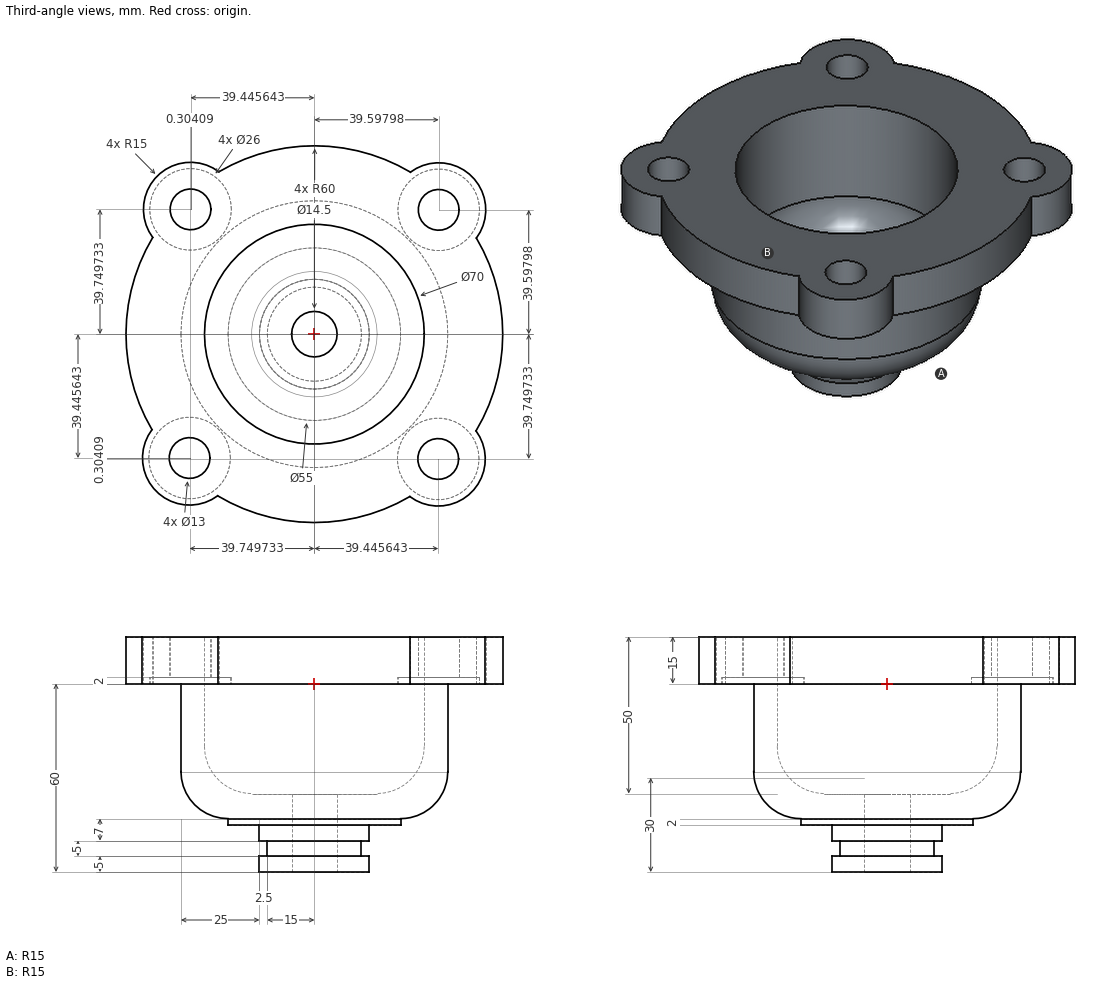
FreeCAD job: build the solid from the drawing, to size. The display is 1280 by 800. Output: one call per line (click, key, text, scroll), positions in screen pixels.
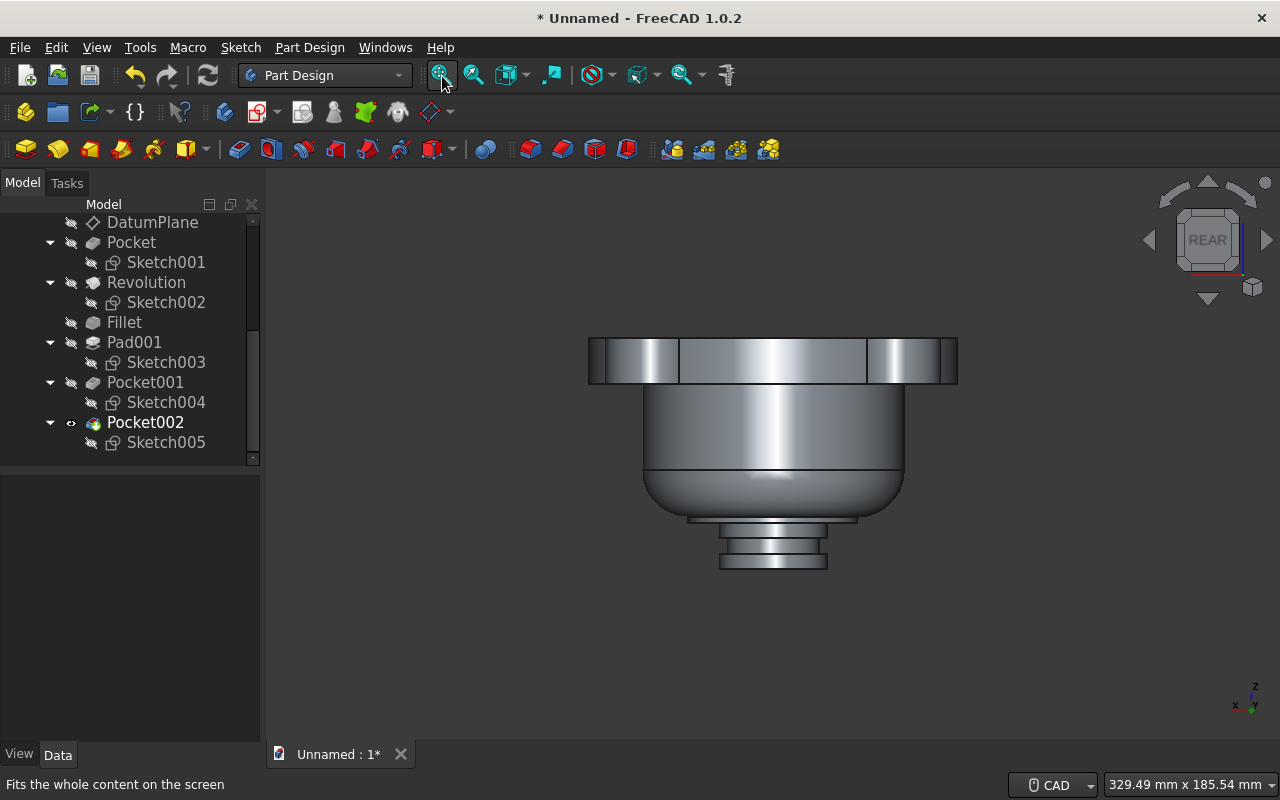
key(6)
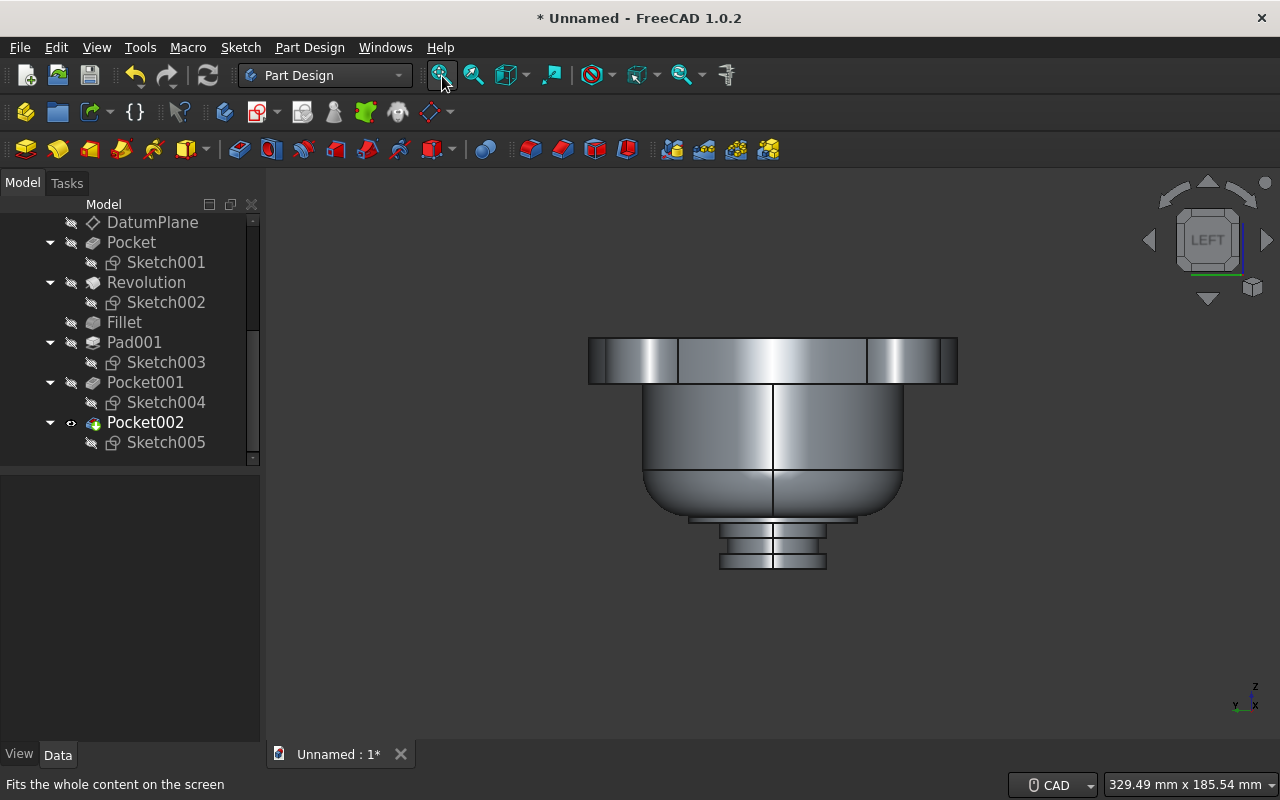
click(442, 76)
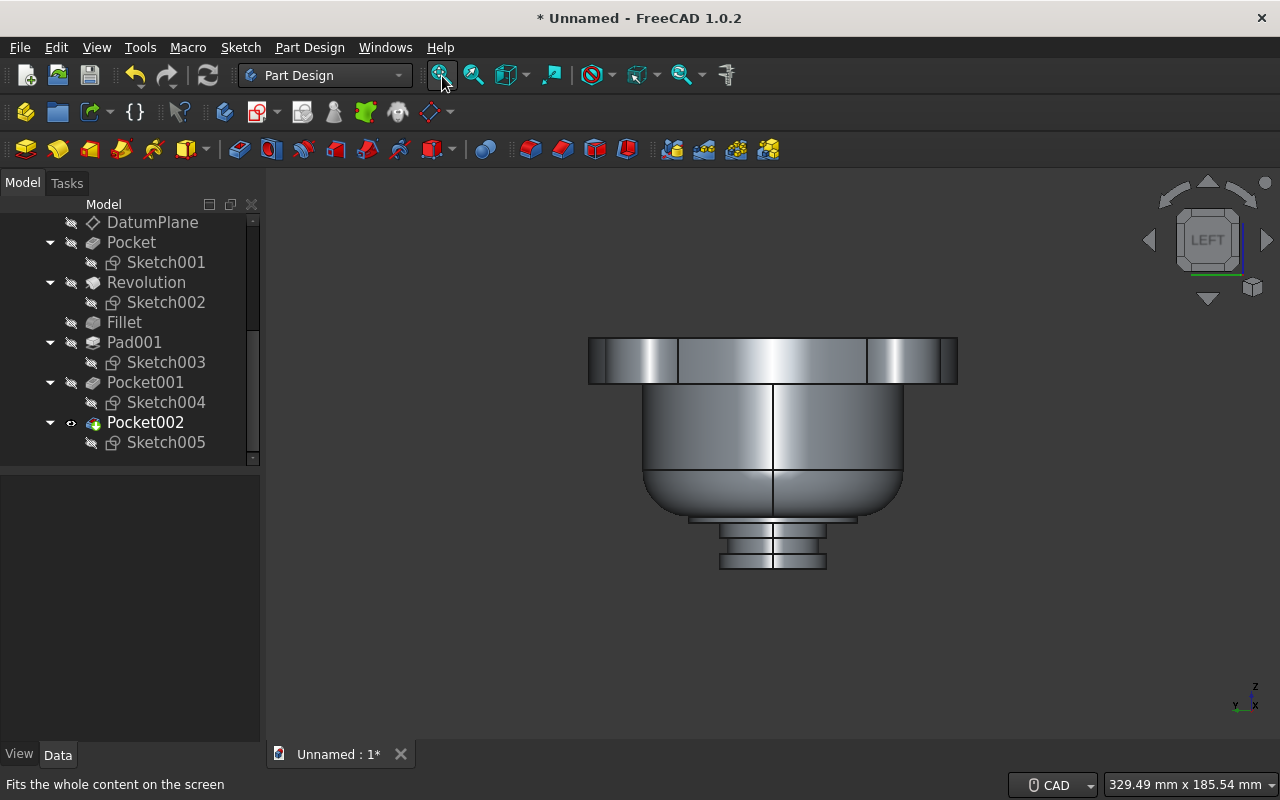
key(v)
key(3)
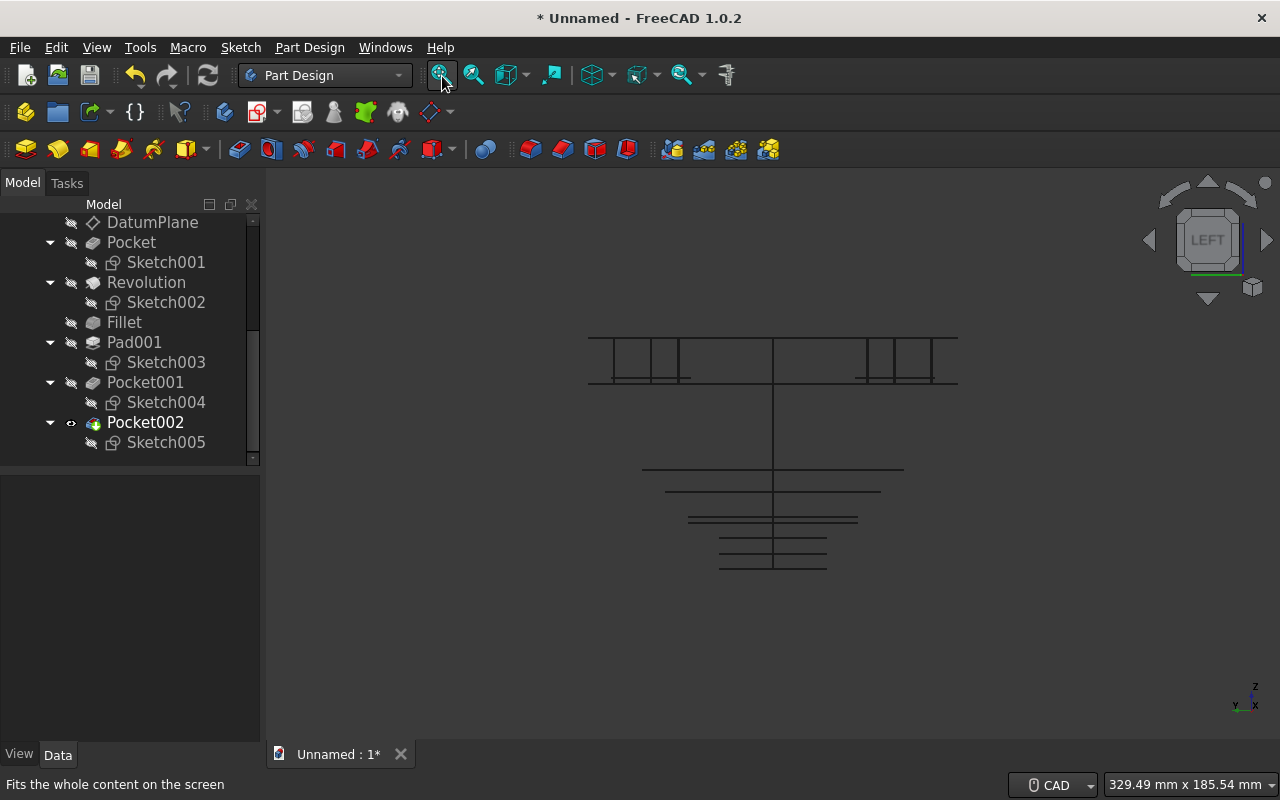
key(0)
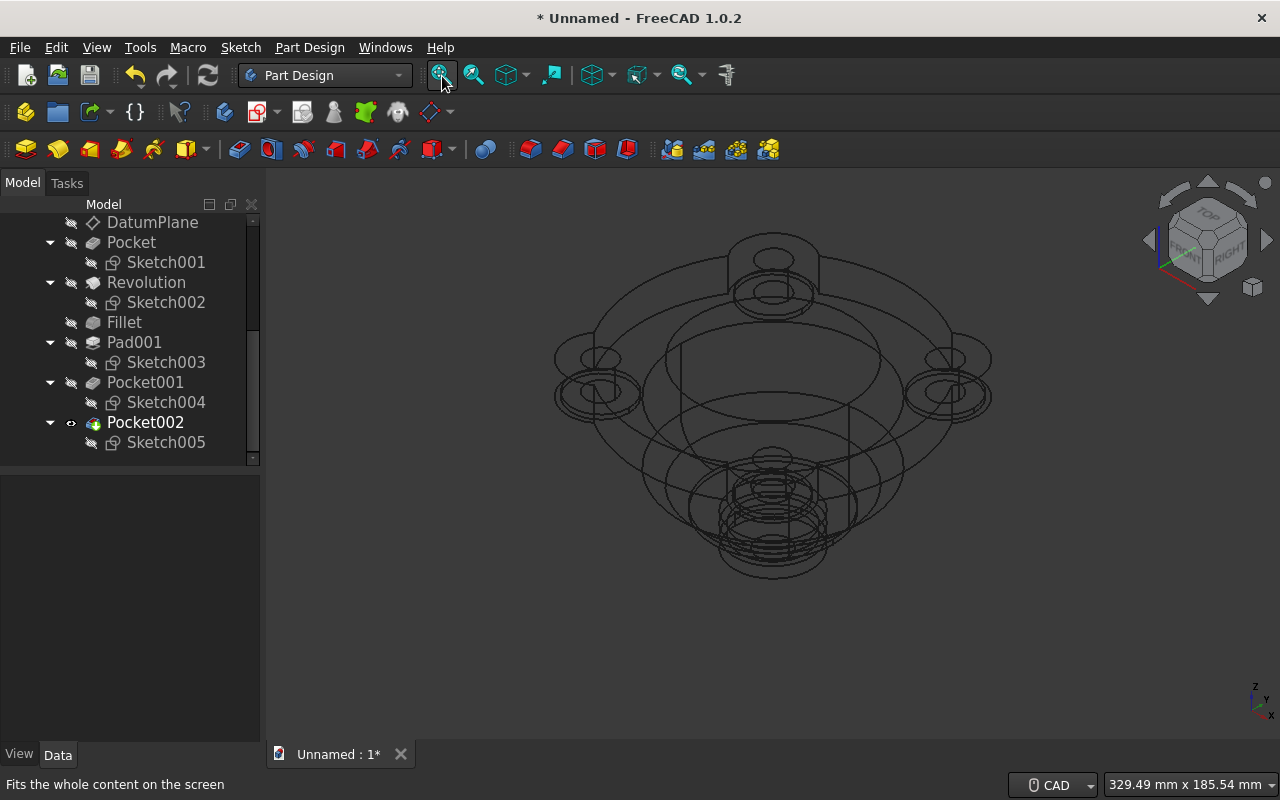
click(697, 440)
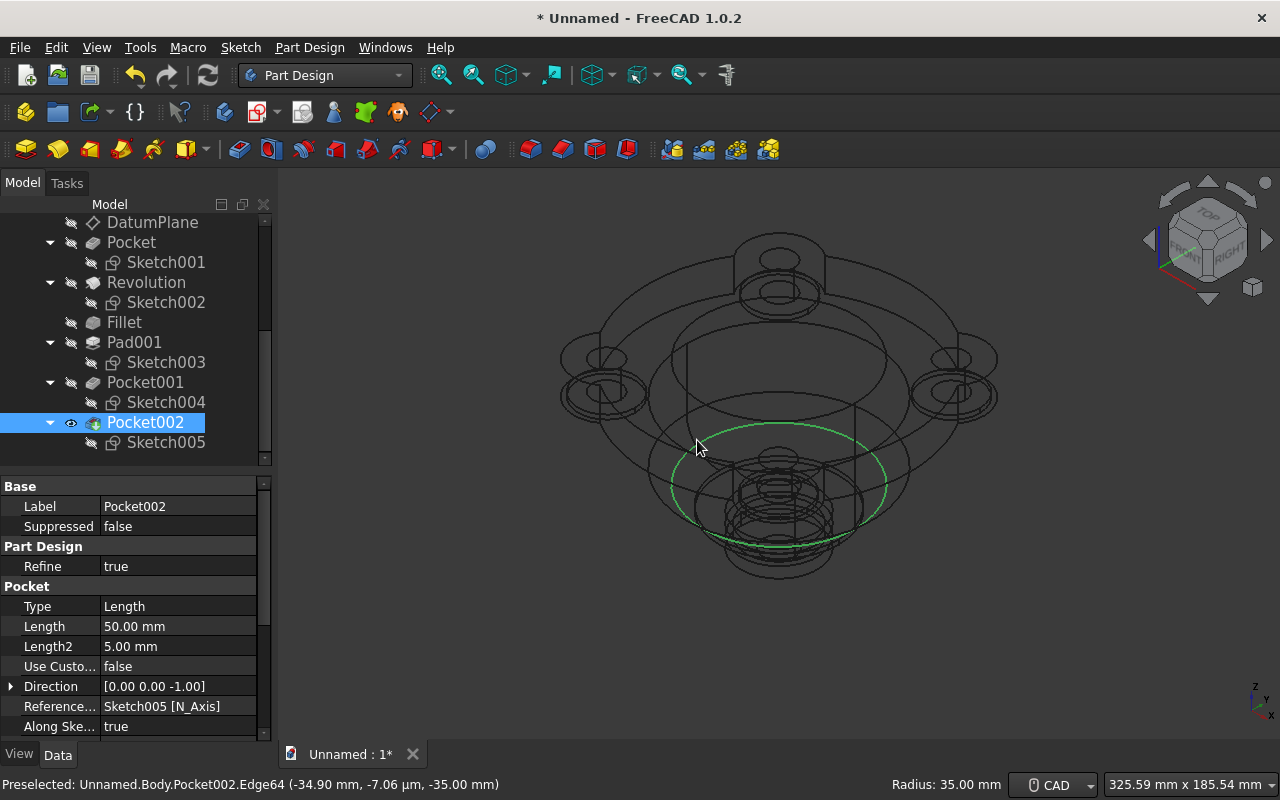
key(v)
key(1)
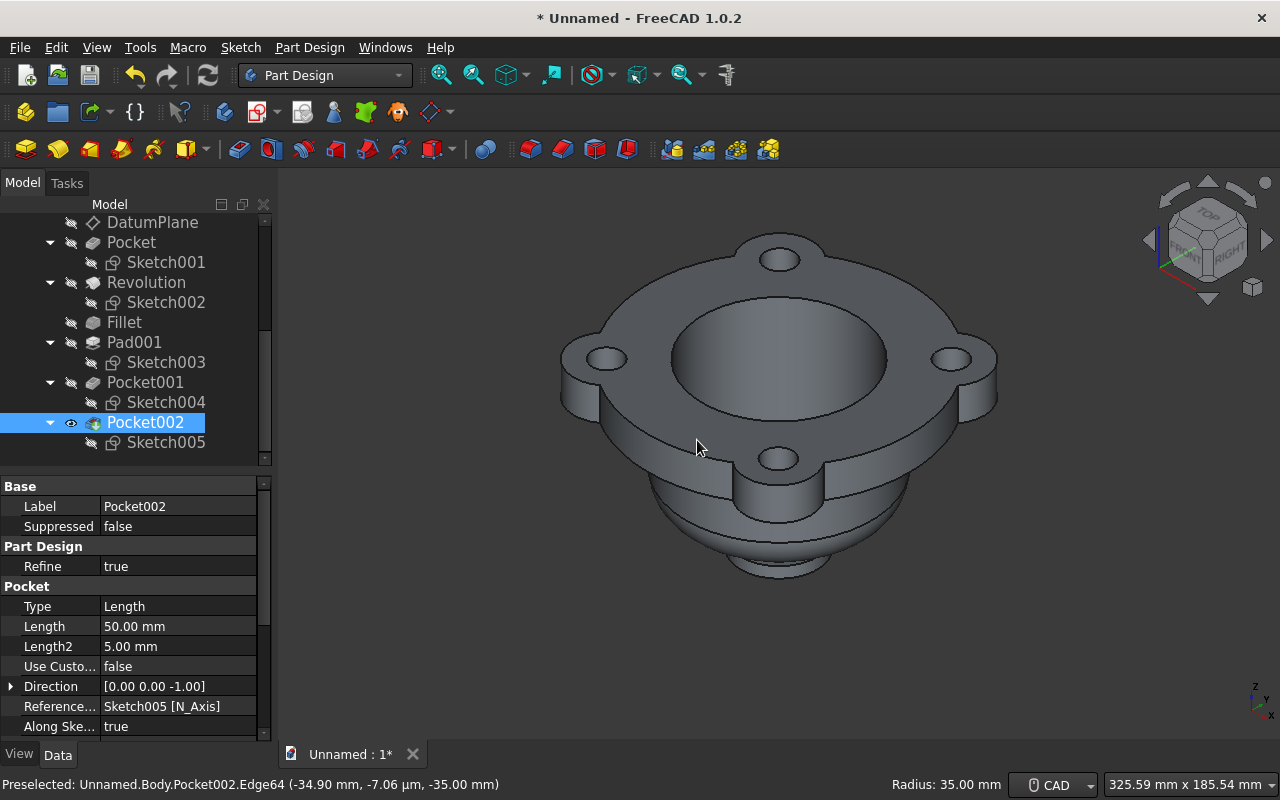
click(532, 150)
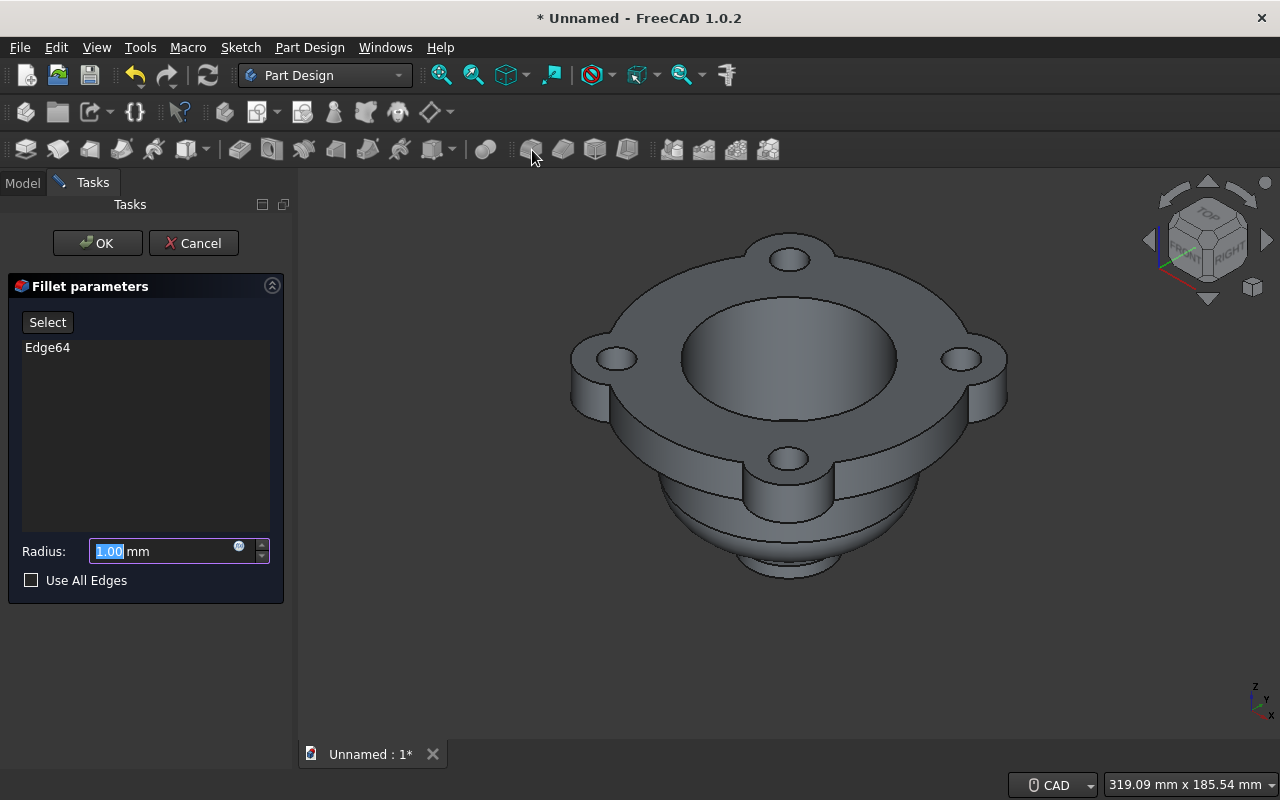
text(15)
key(Tab)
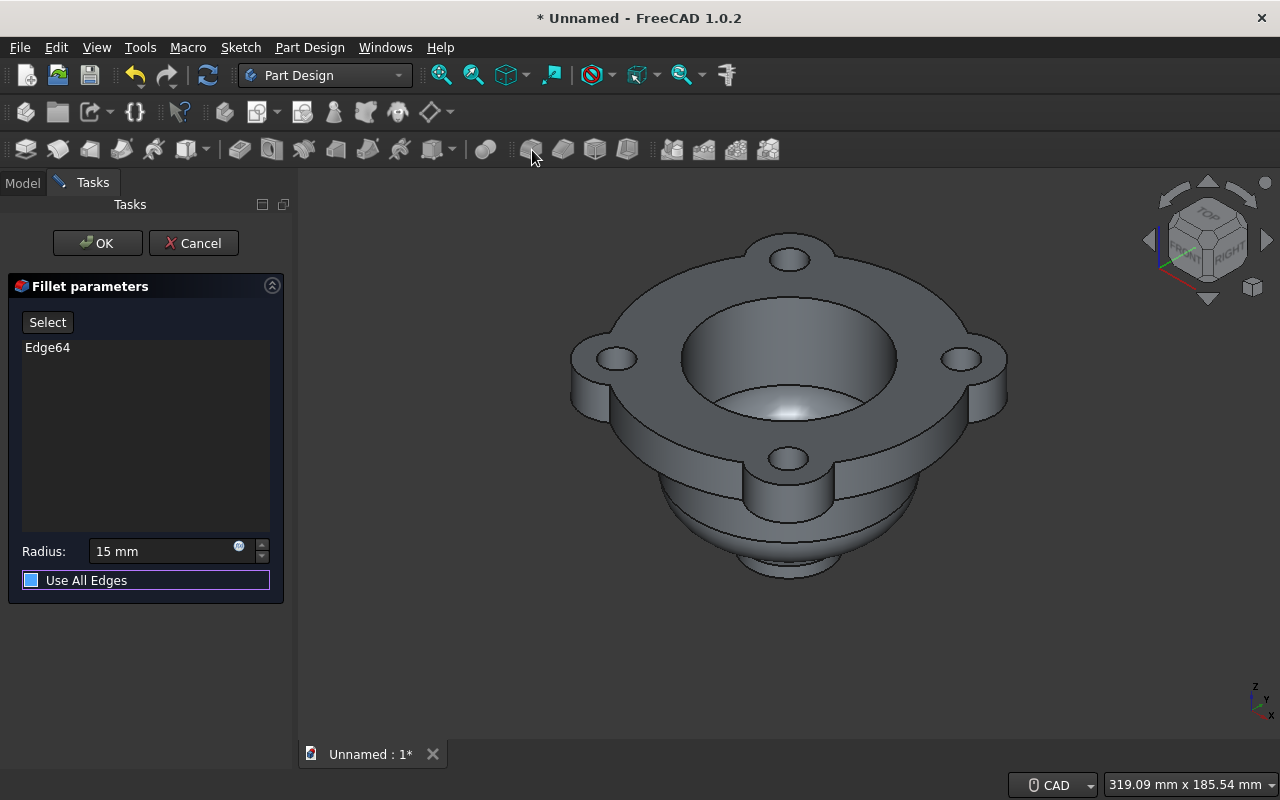
click(98, 243)